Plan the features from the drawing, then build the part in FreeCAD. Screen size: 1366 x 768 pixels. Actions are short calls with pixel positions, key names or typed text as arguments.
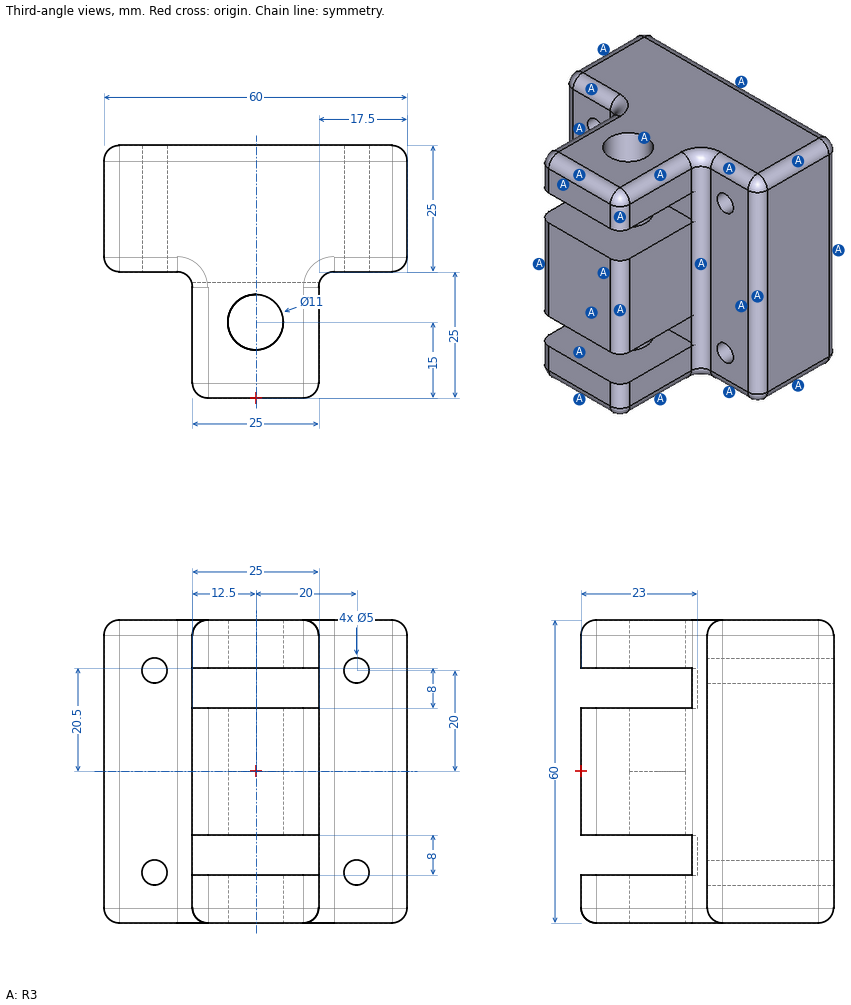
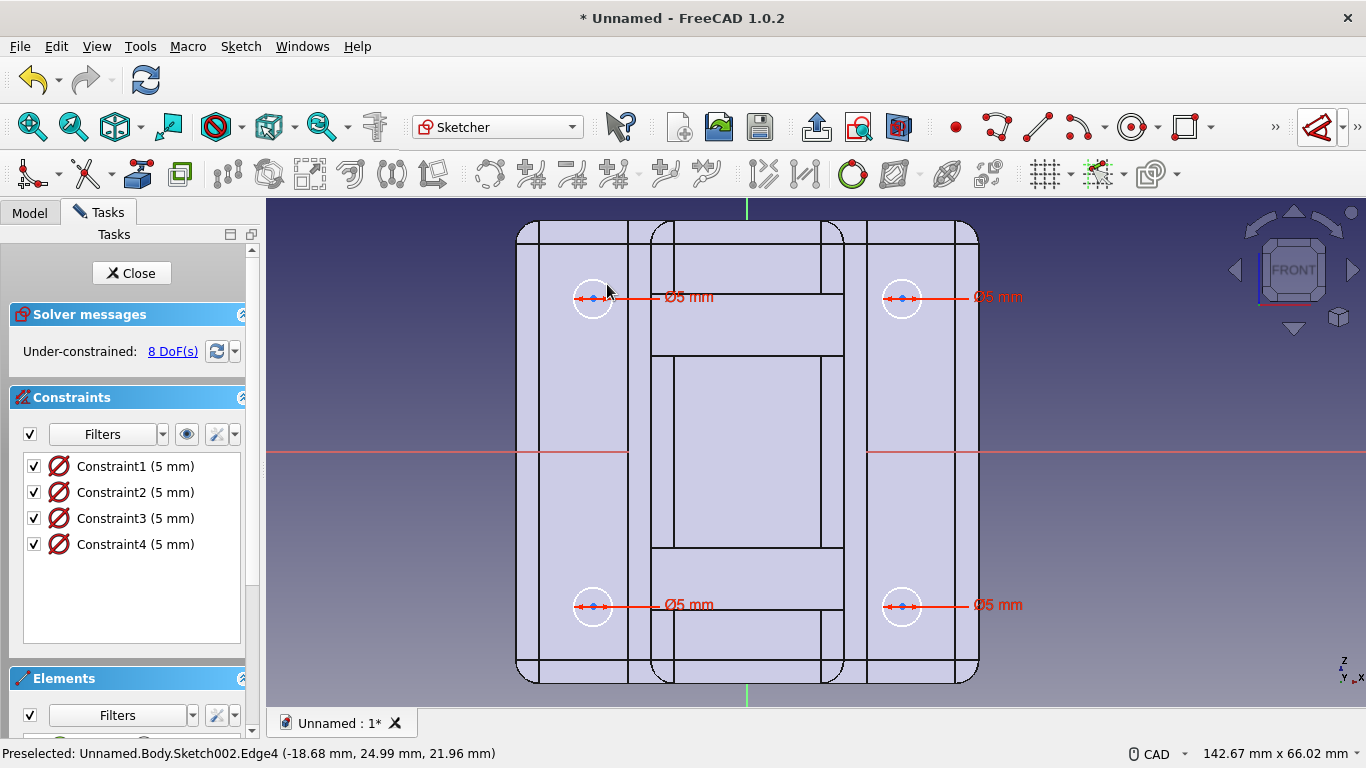
click(902, 299)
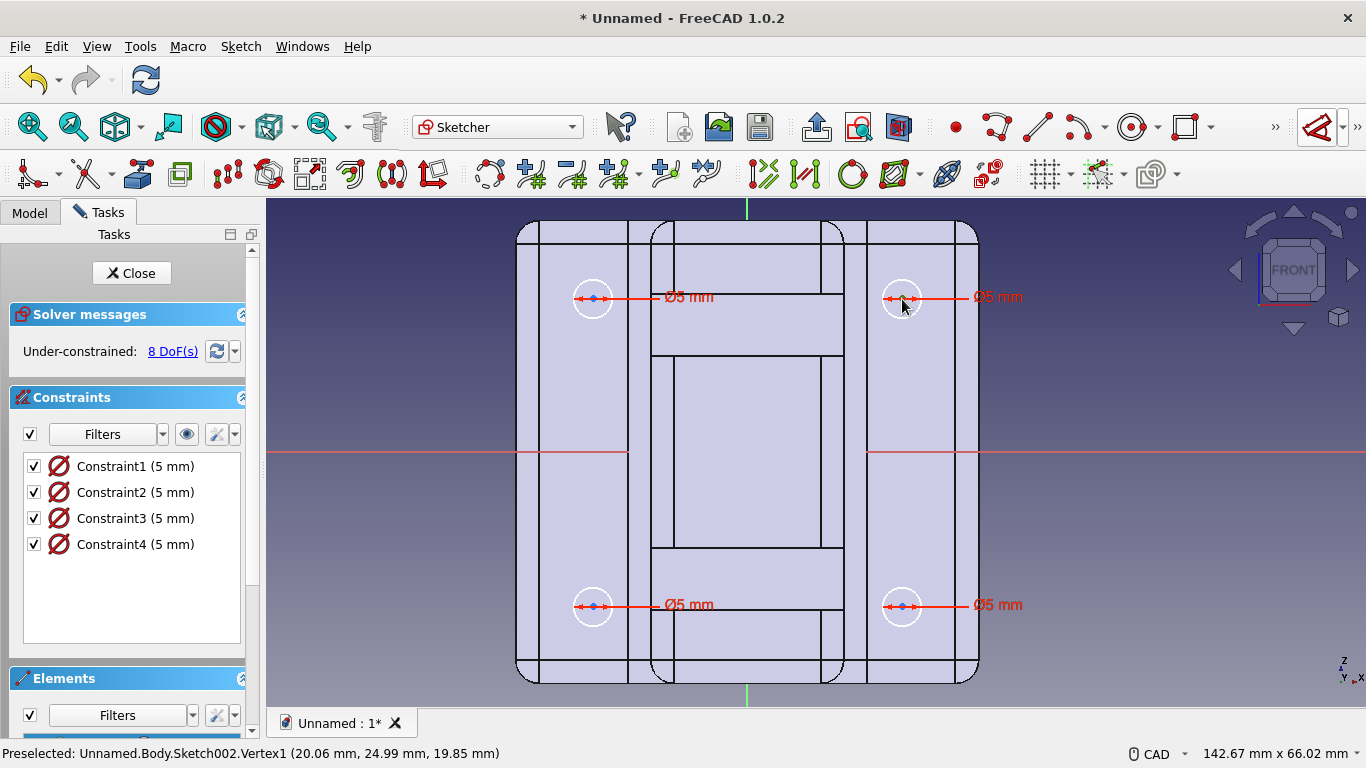
click(902, 607)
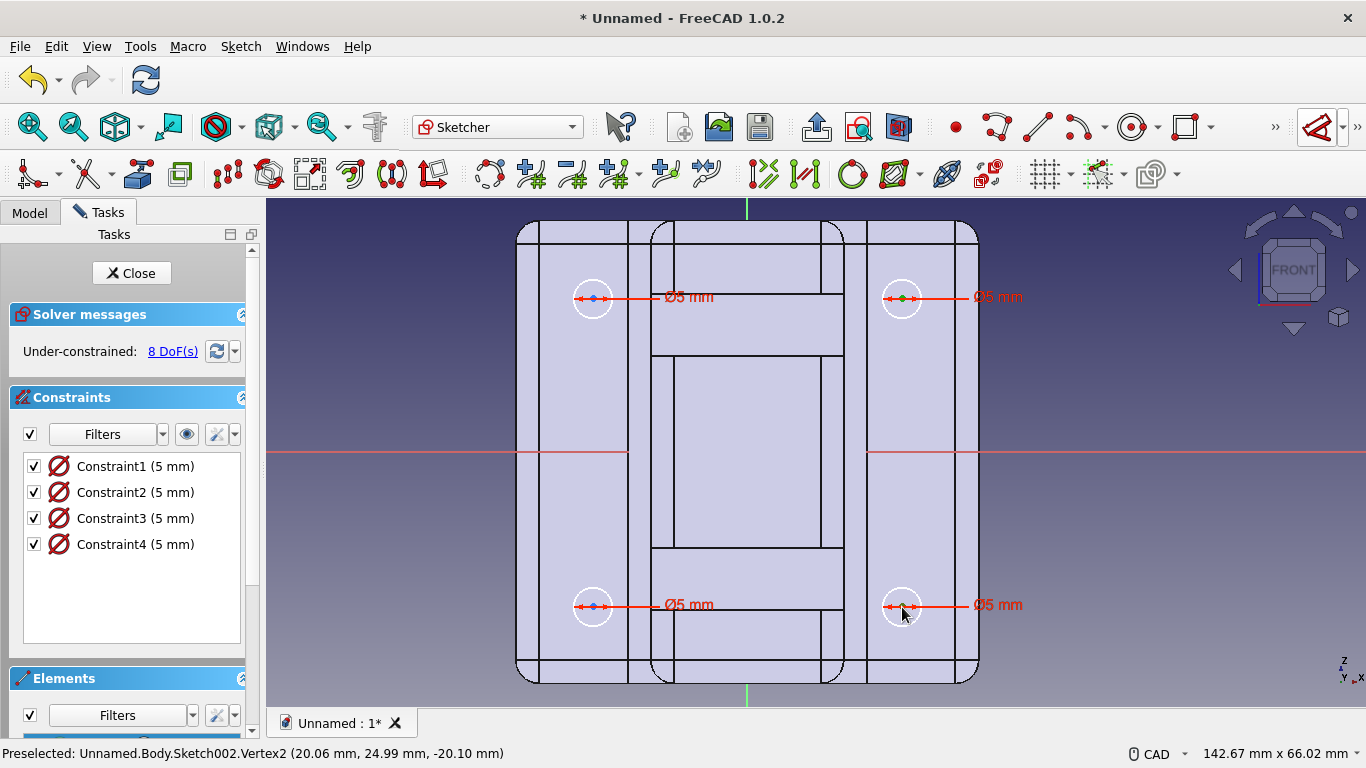
click(359, 452)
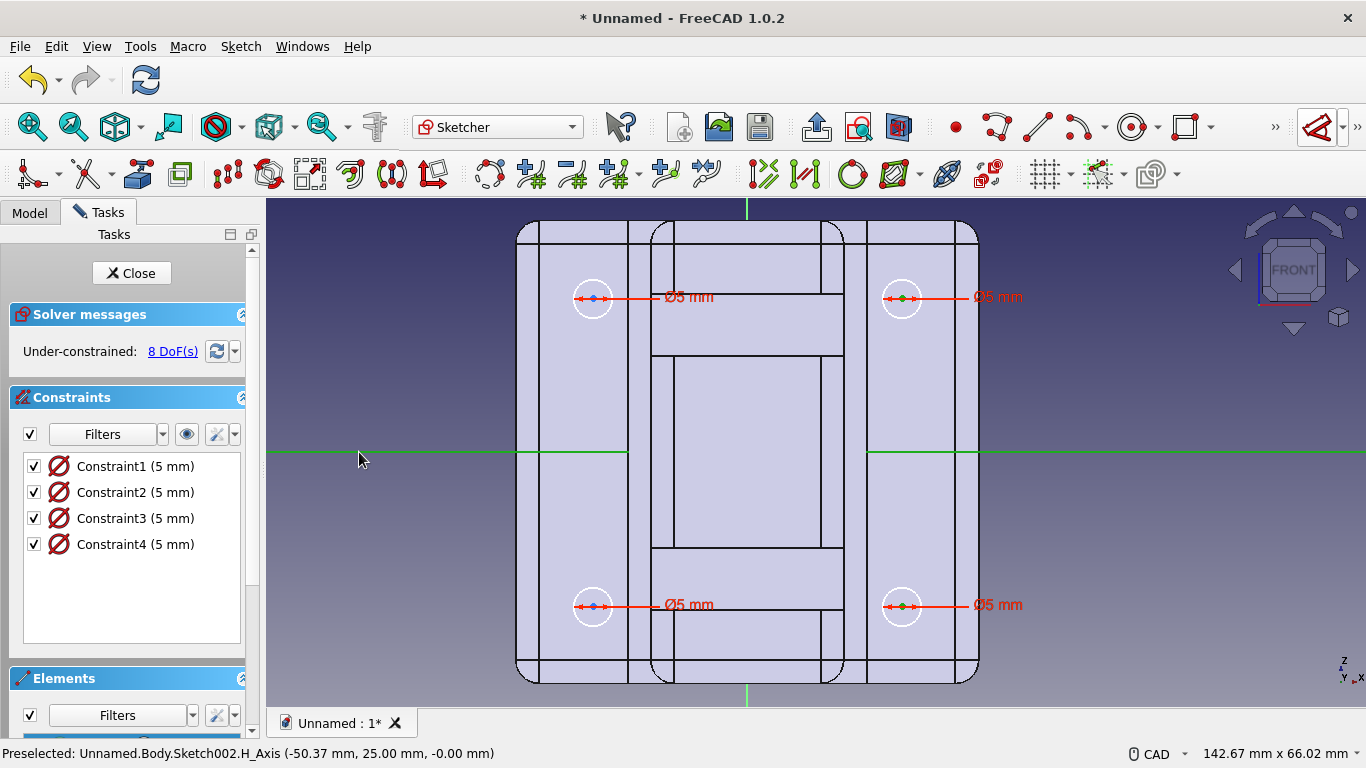
key(s)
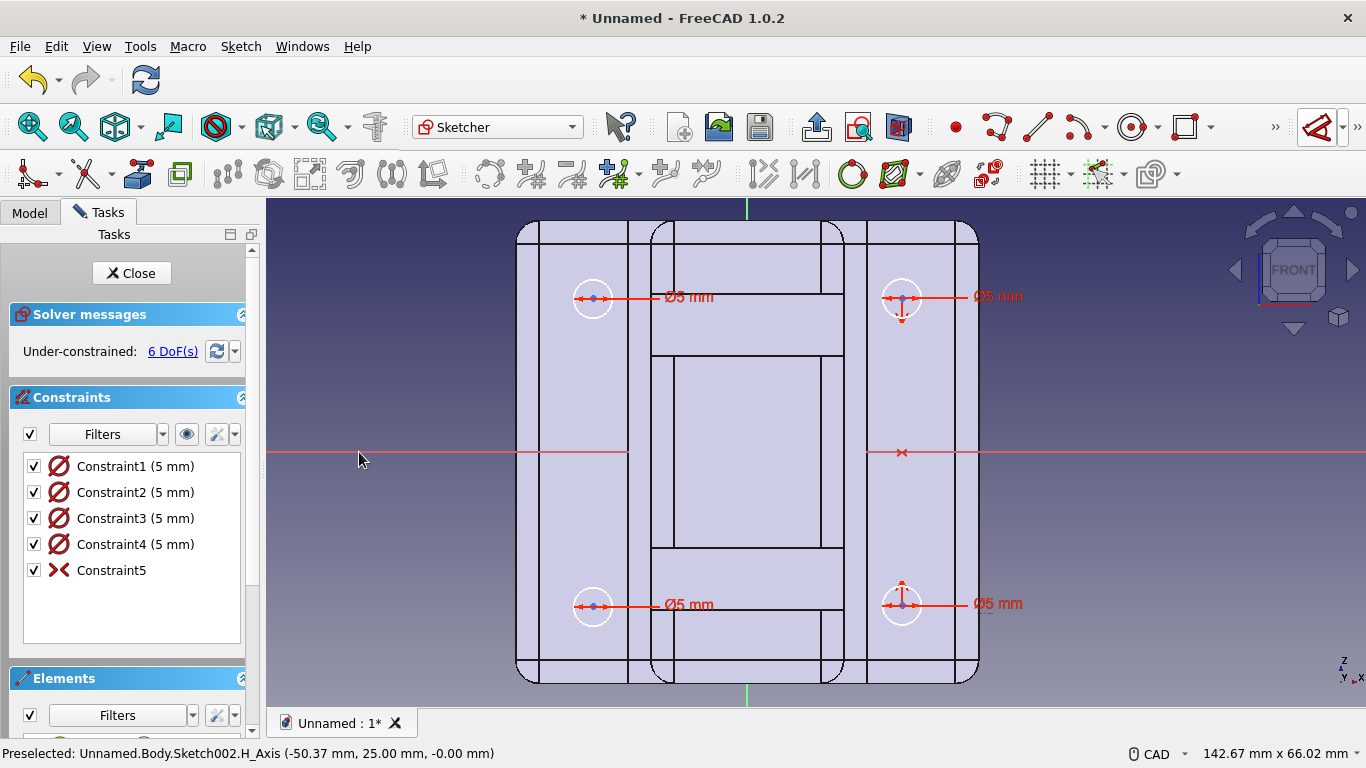
click(902, 606)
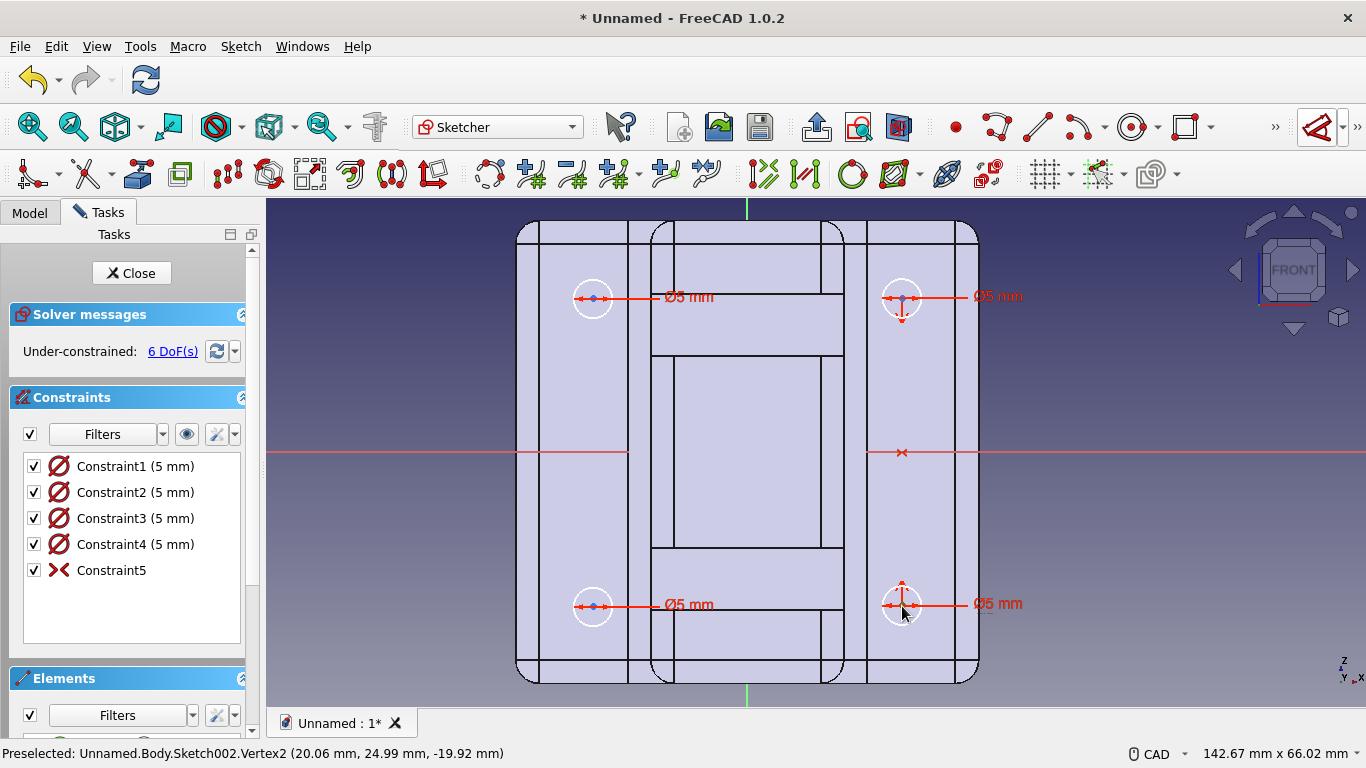
click(593, 607)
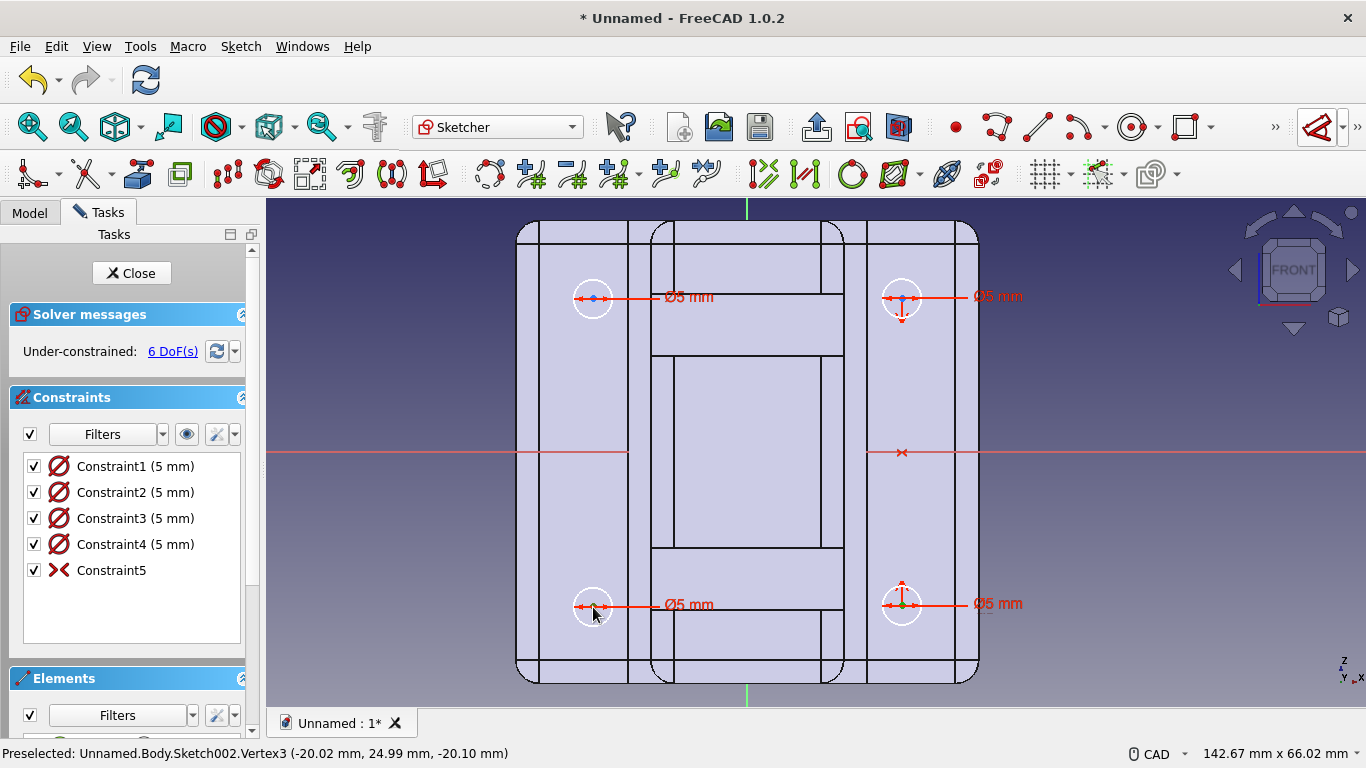
click(747, 647)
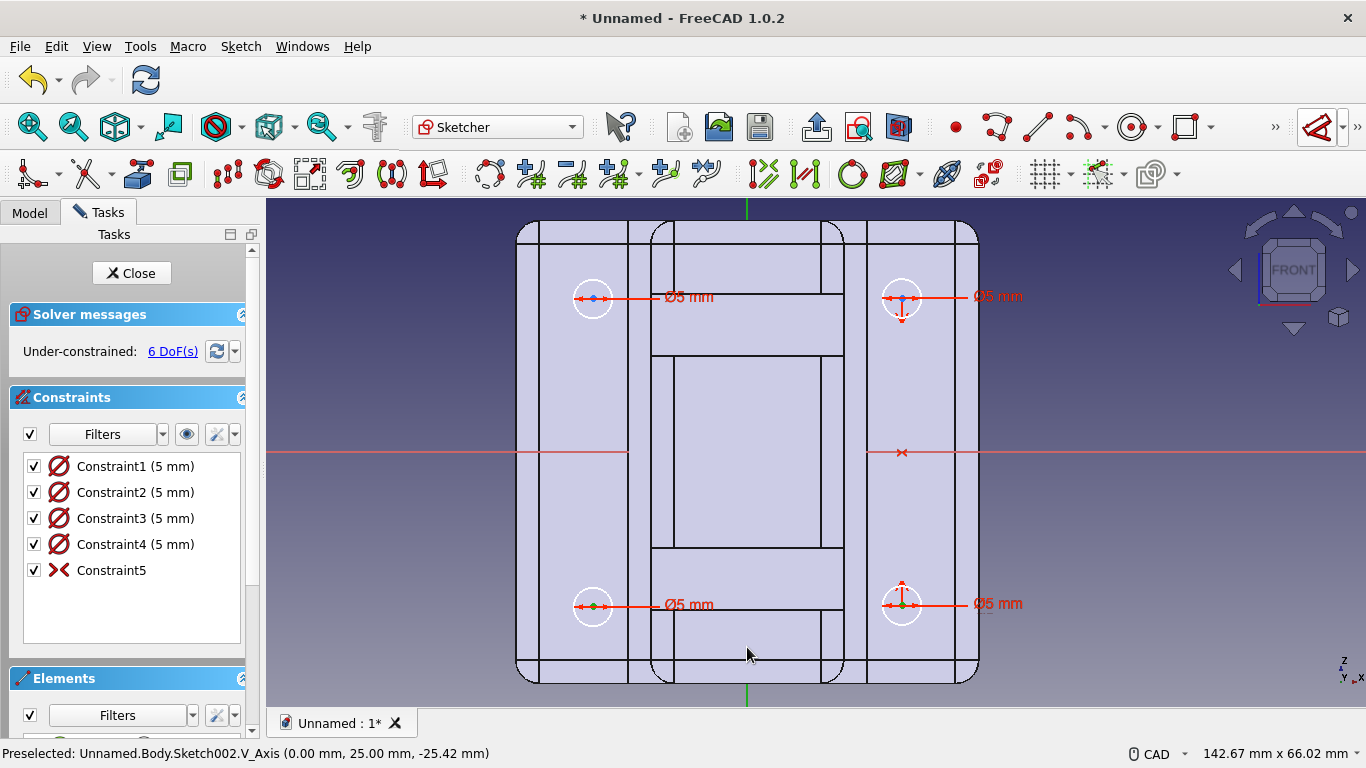
key(s)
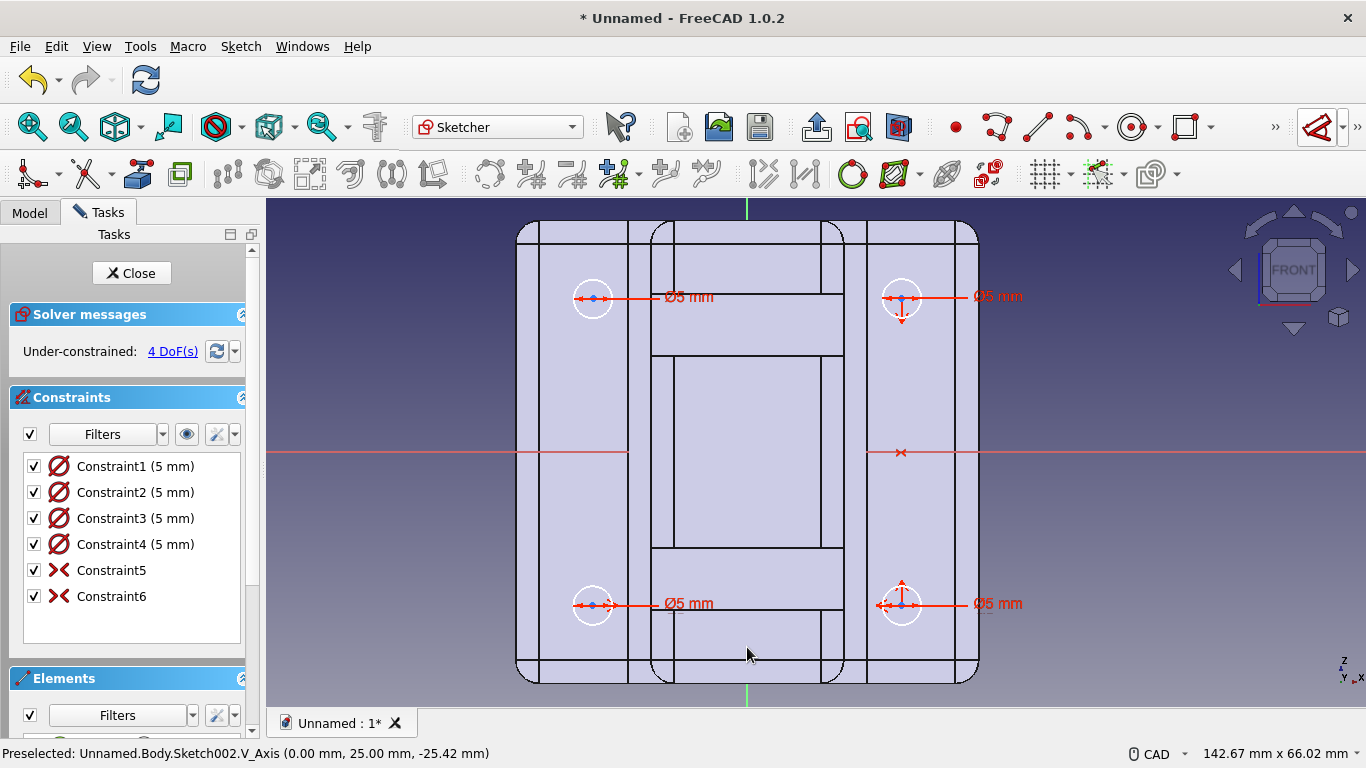
click(902, 298)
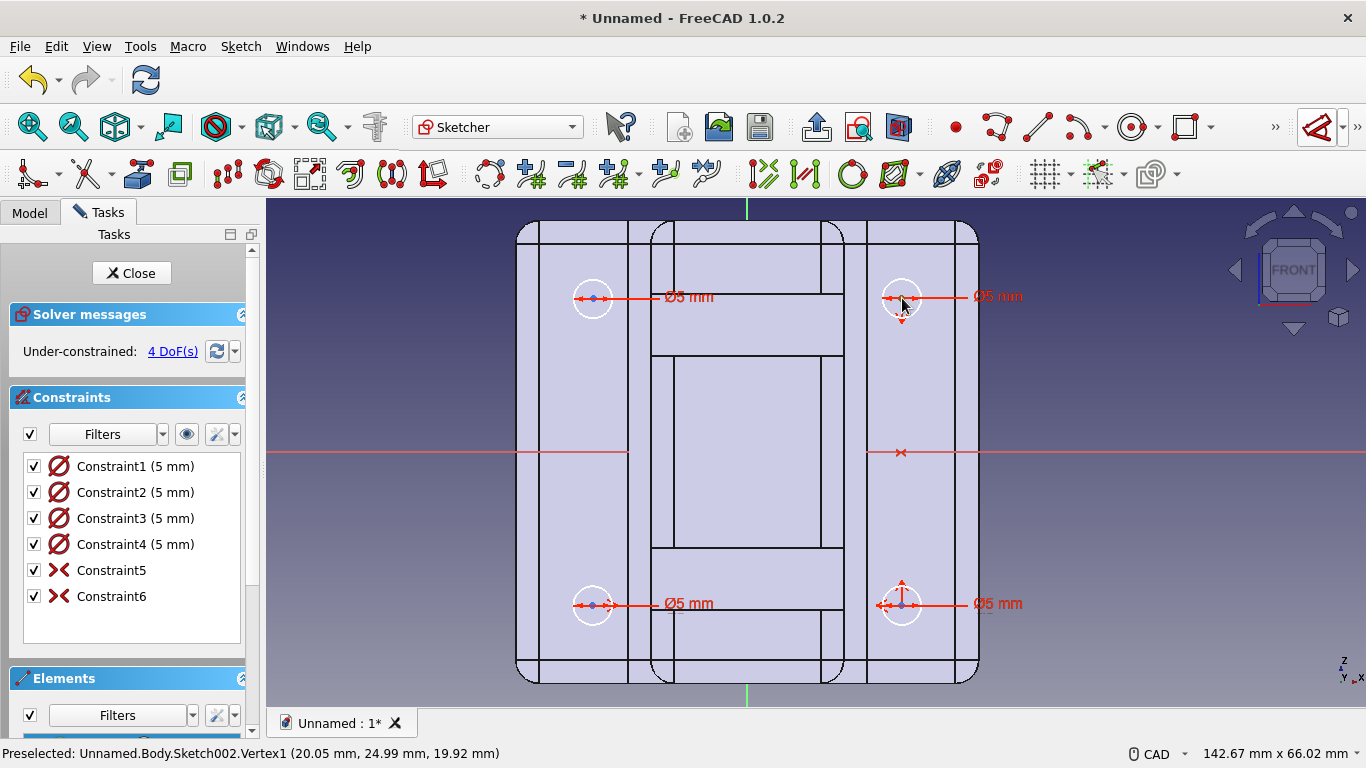
click(593, 299)